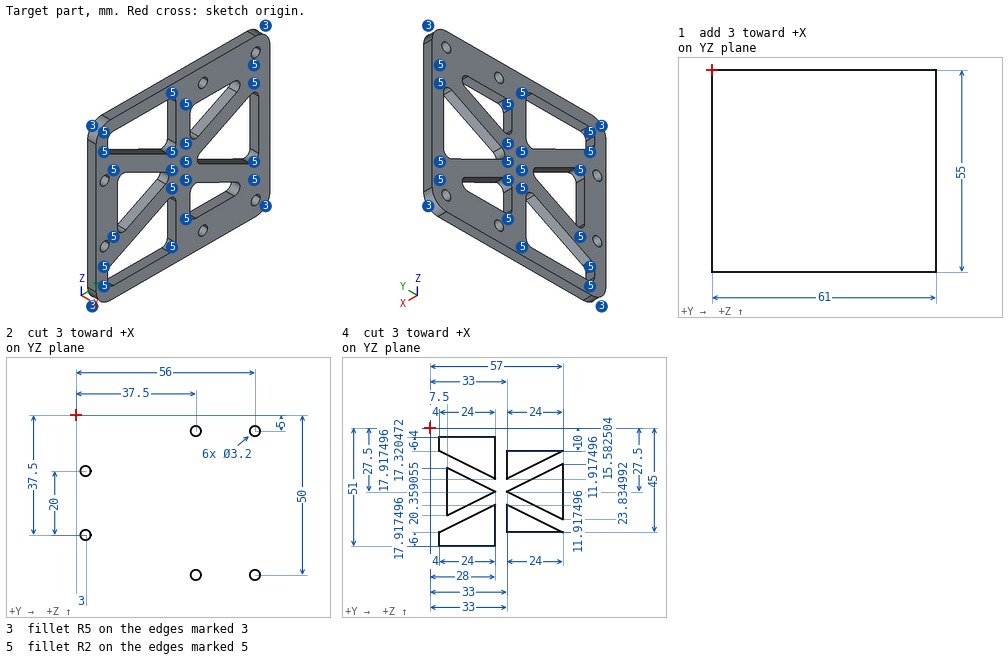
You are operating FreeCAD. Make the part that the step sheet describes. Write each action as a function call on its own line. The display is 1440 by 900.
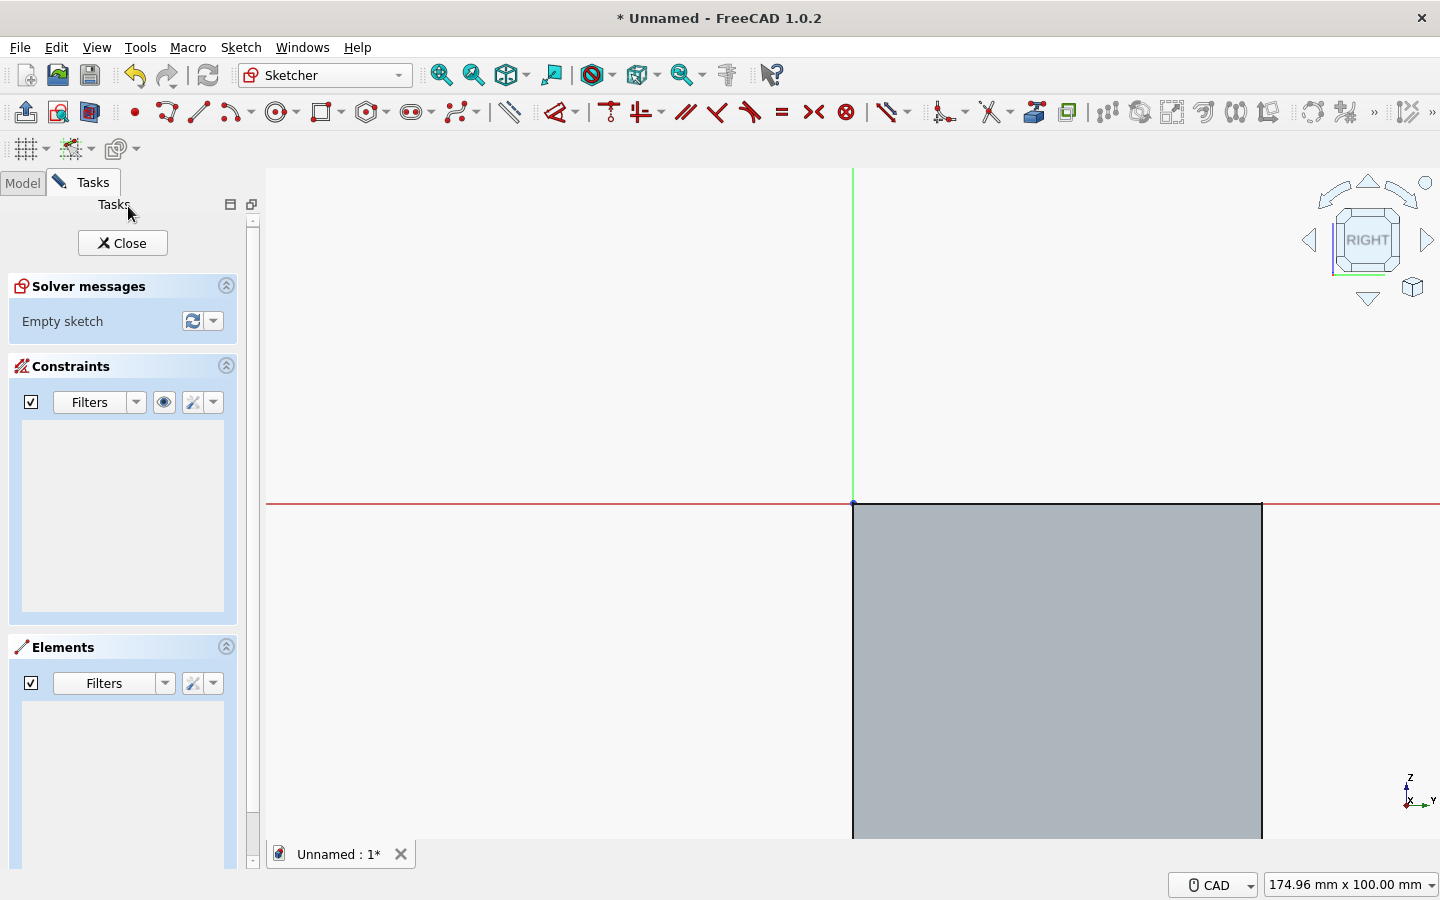
click(90, 112)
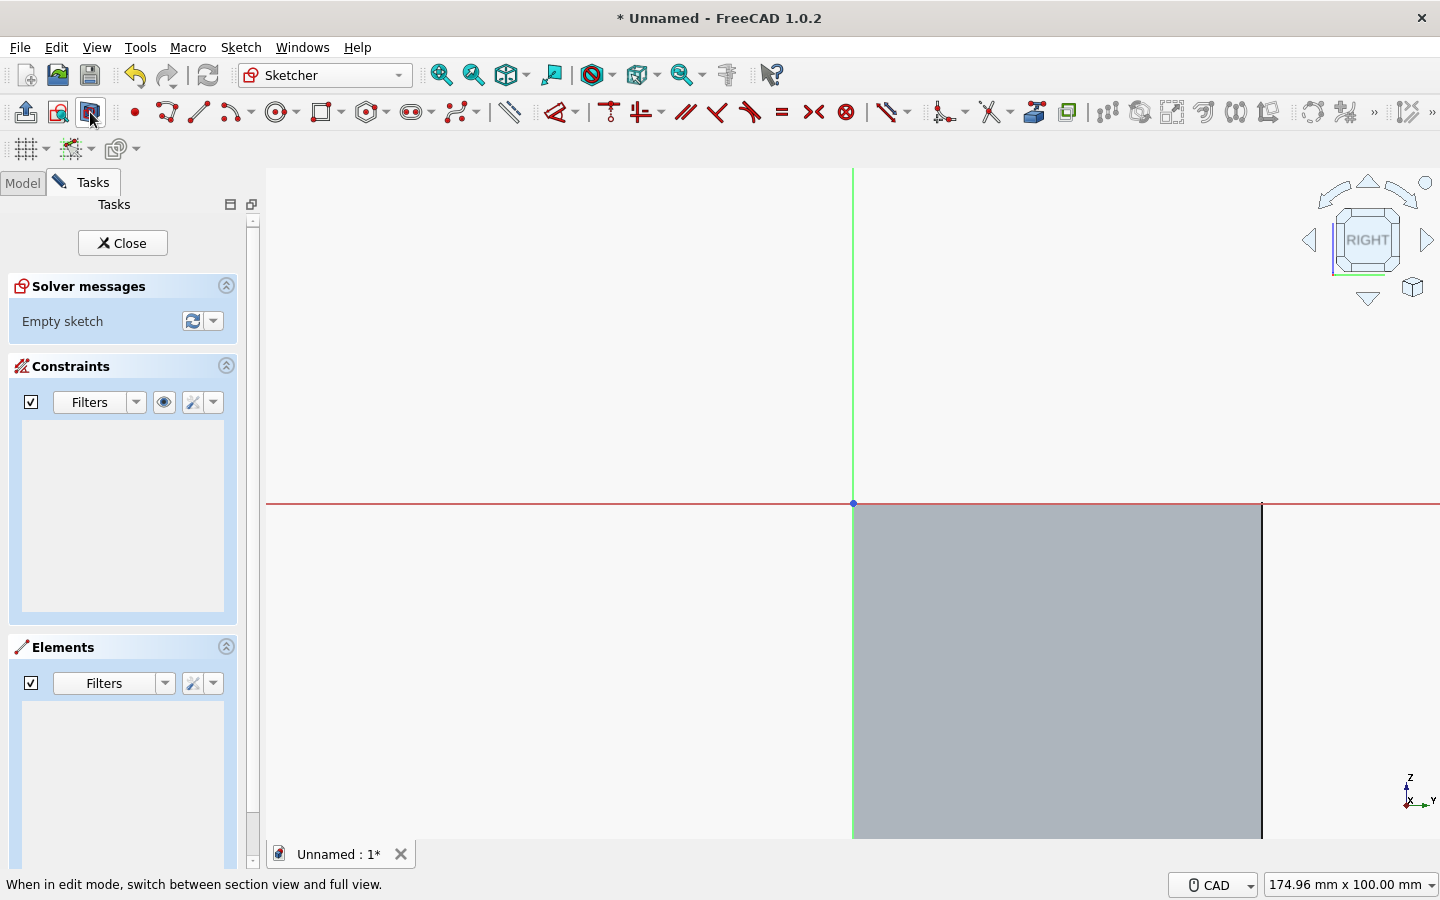
scroll(294, 196, down, 1)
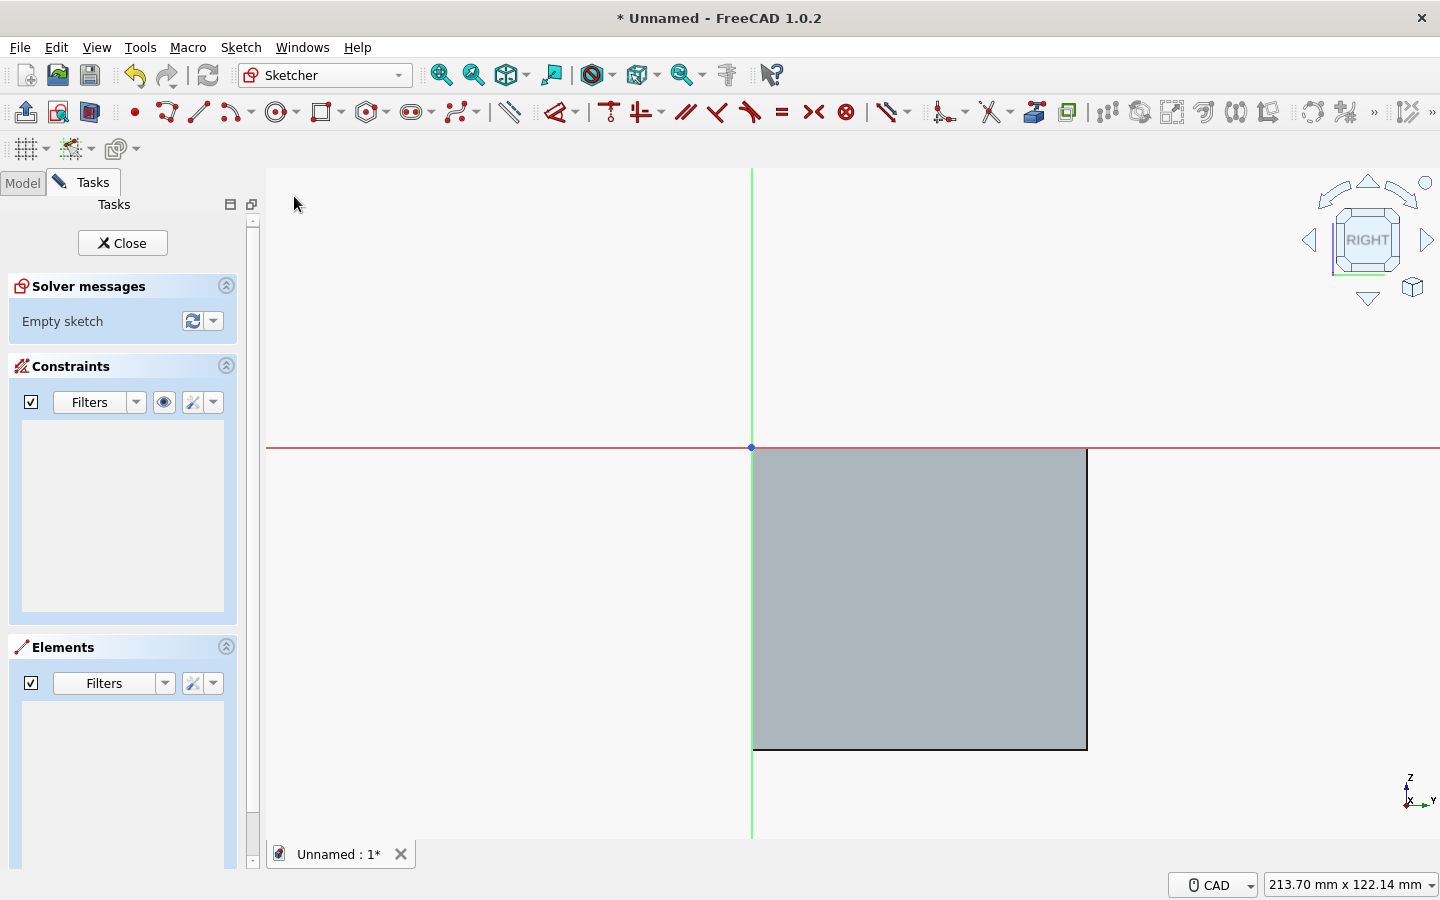
scroll(1165, 764, up, 2)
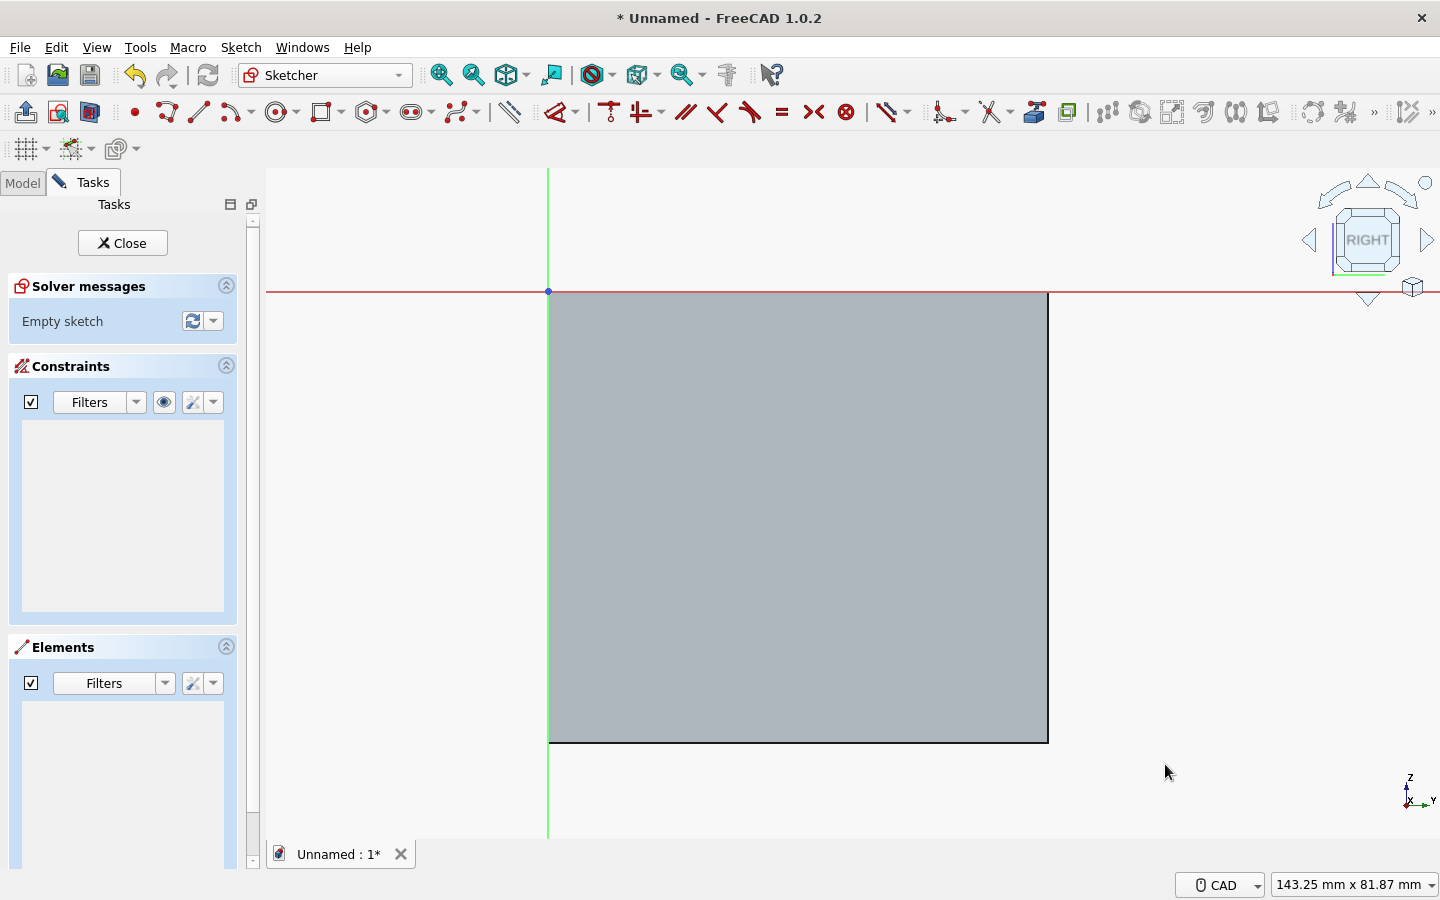
click(276, 112)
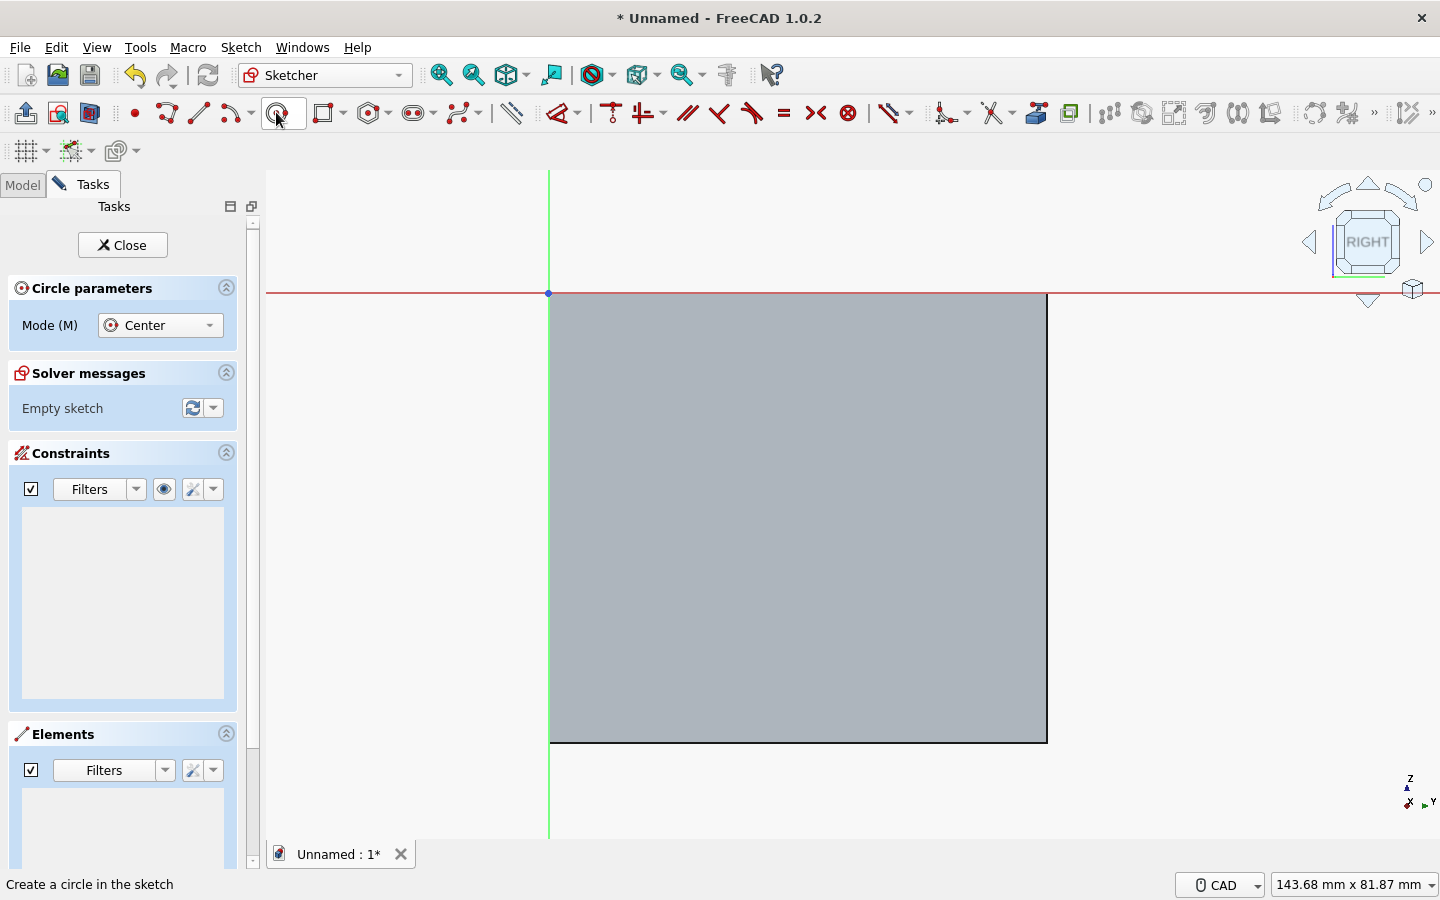
scroll(1007, 334, up, 3)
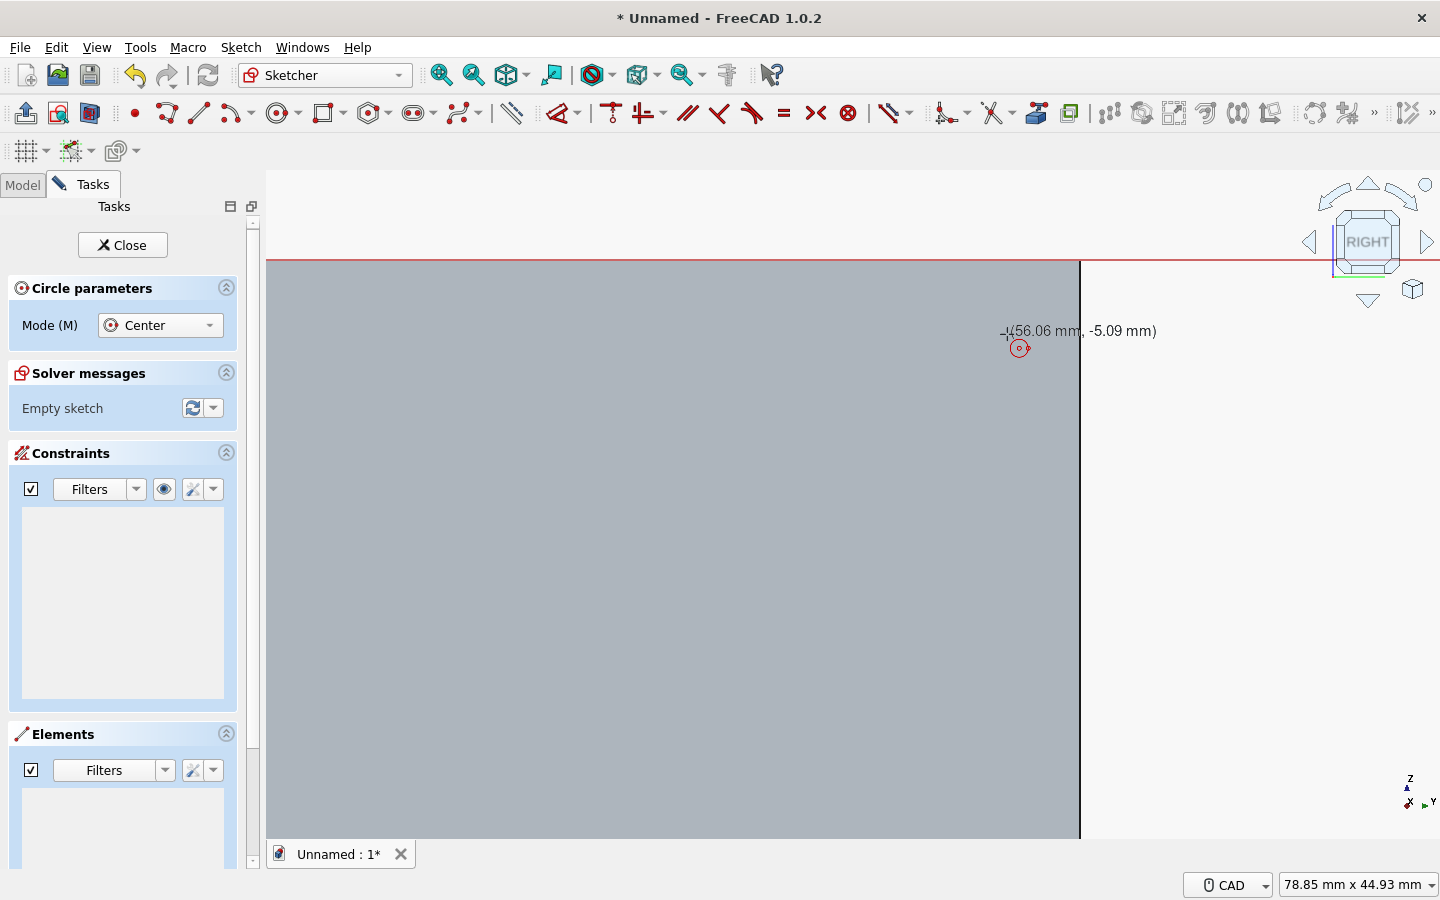
click(1006, 334)
move(1022, 317)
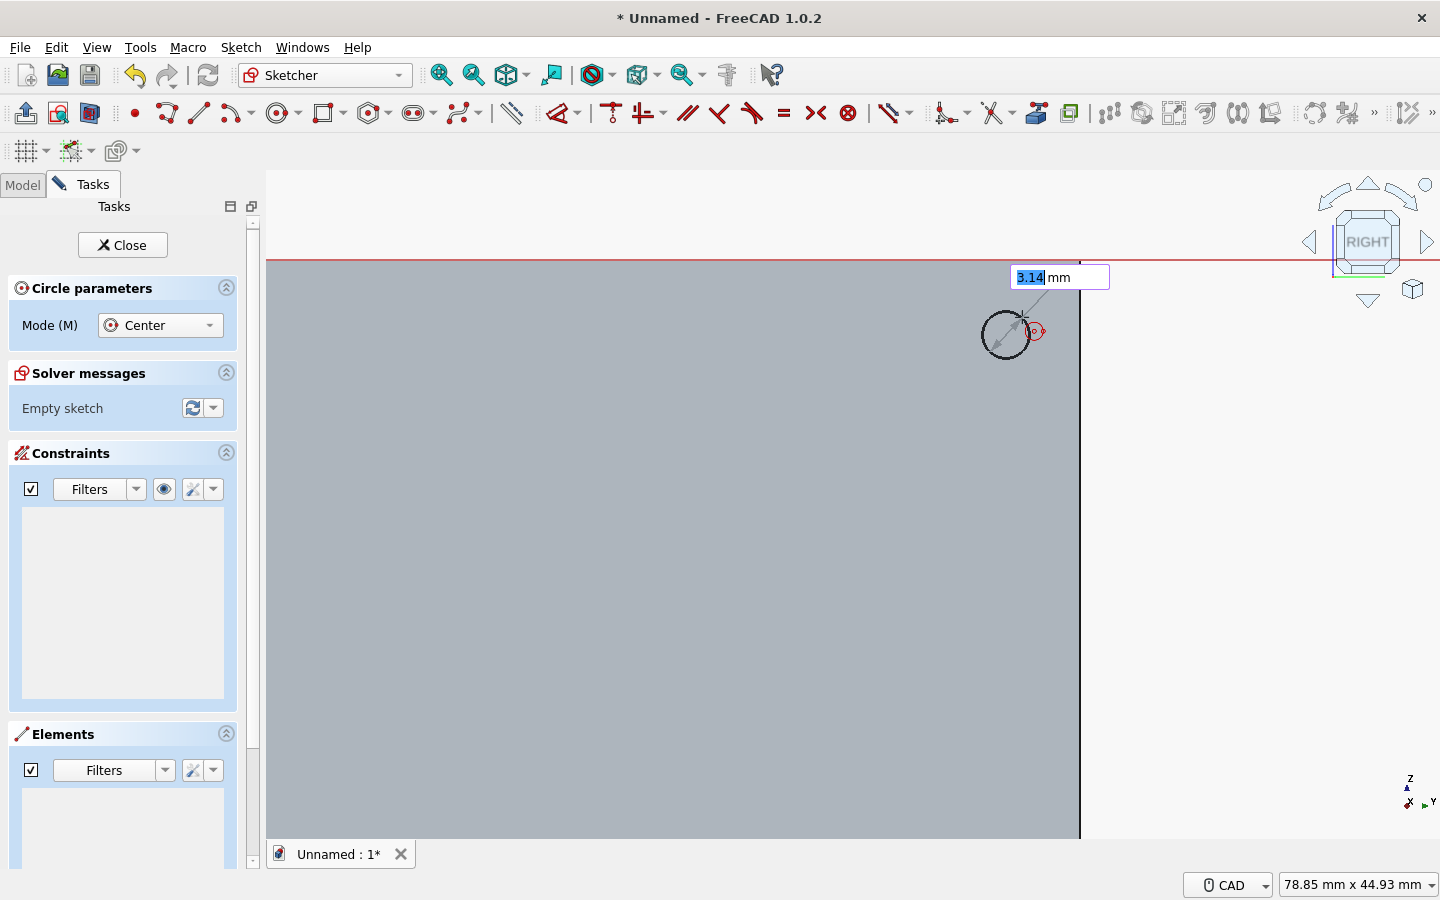
text(3.2)
key(Return)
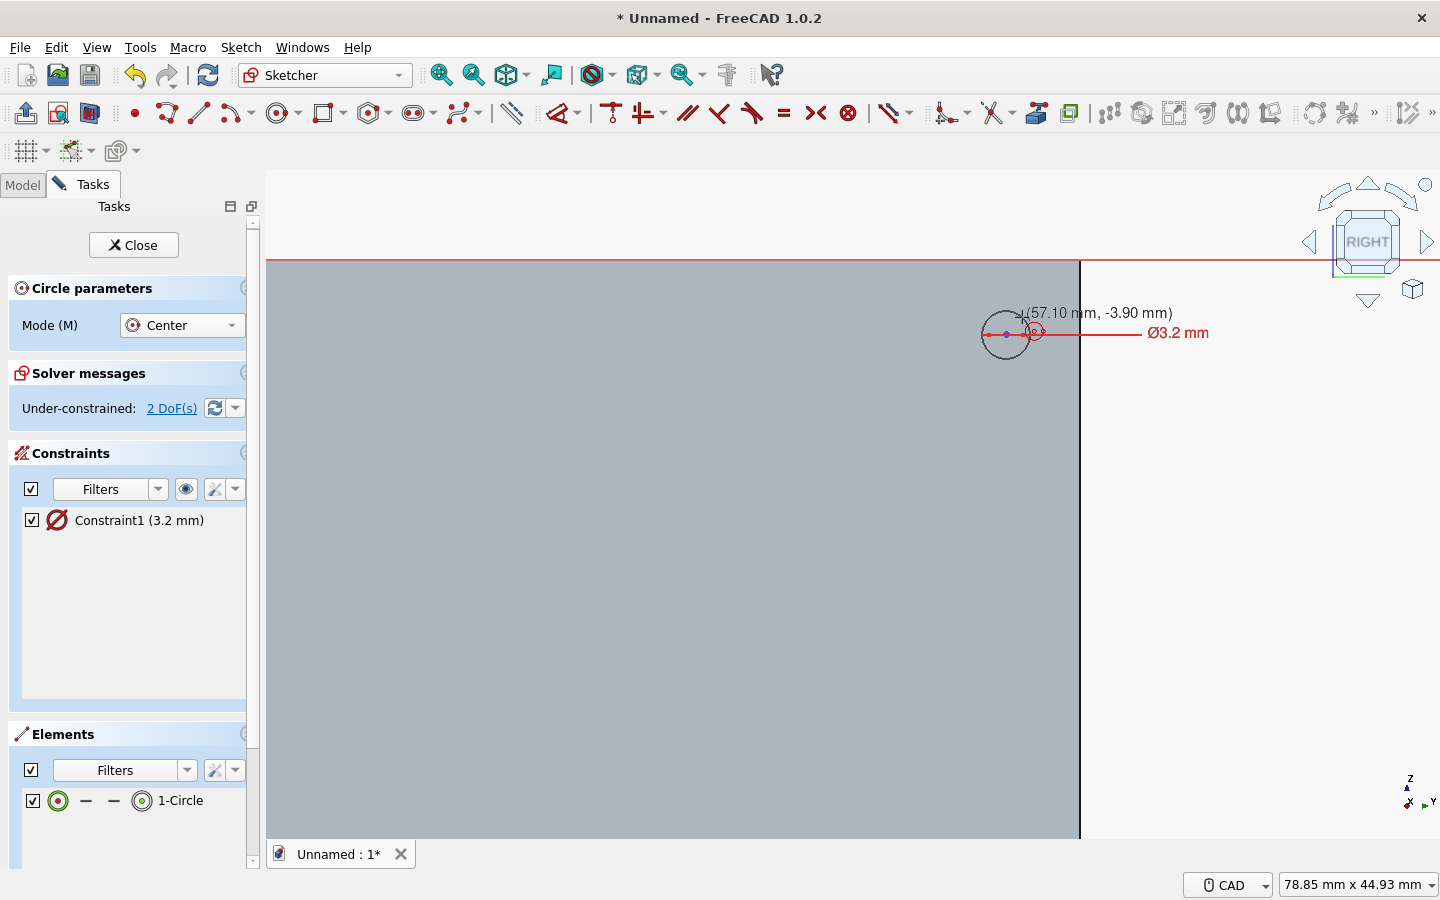
click(730, 334)
move(747, 317)